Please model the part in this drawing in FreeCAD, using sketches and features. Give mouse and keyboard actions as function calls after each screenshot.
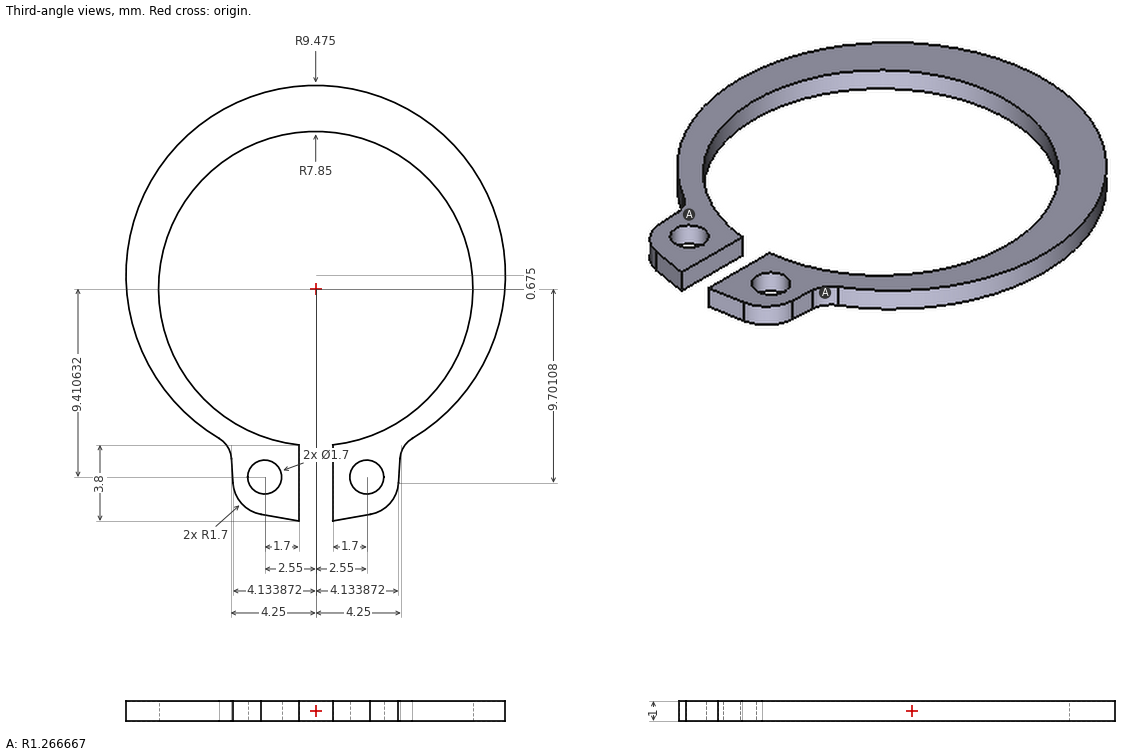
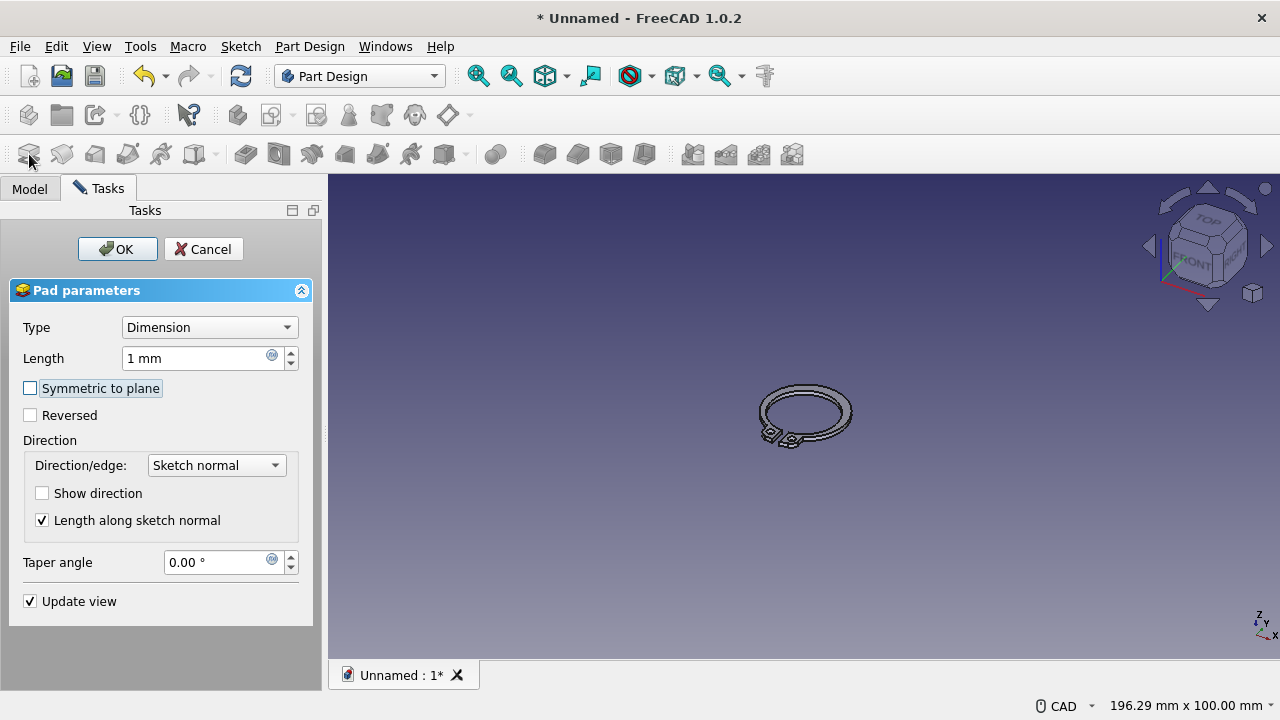
click(31, 388)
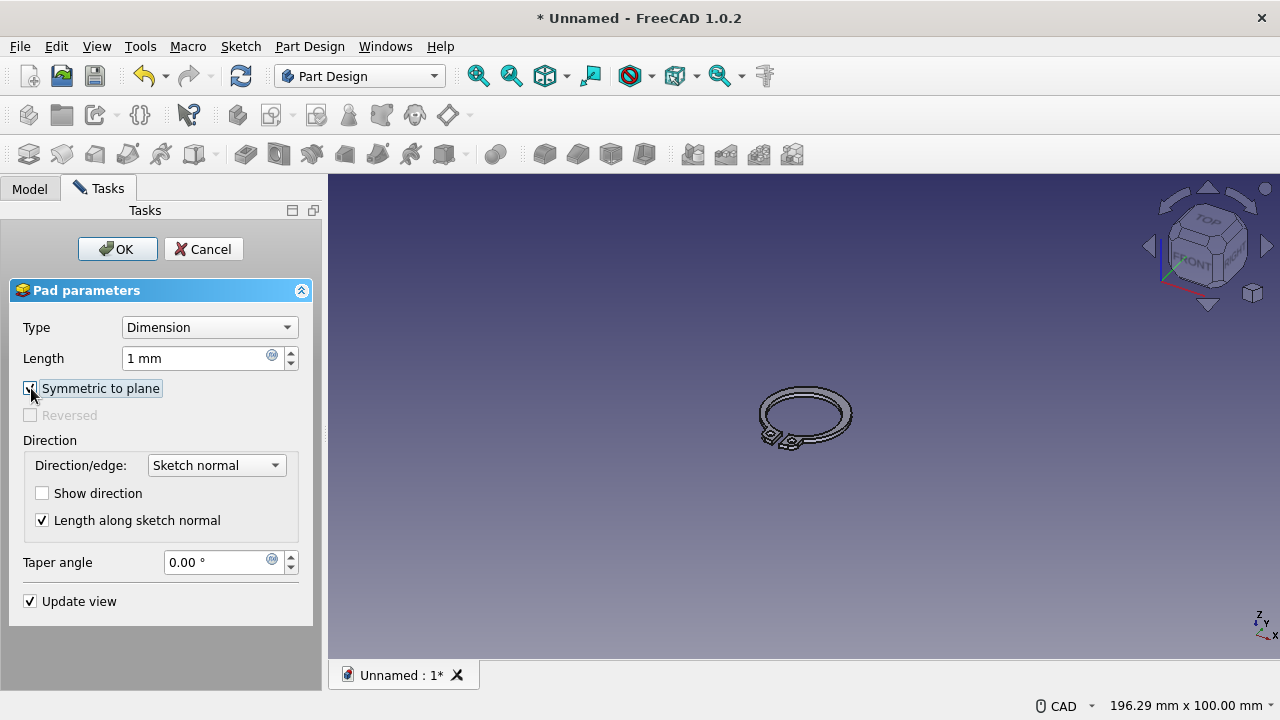
click(118, 249)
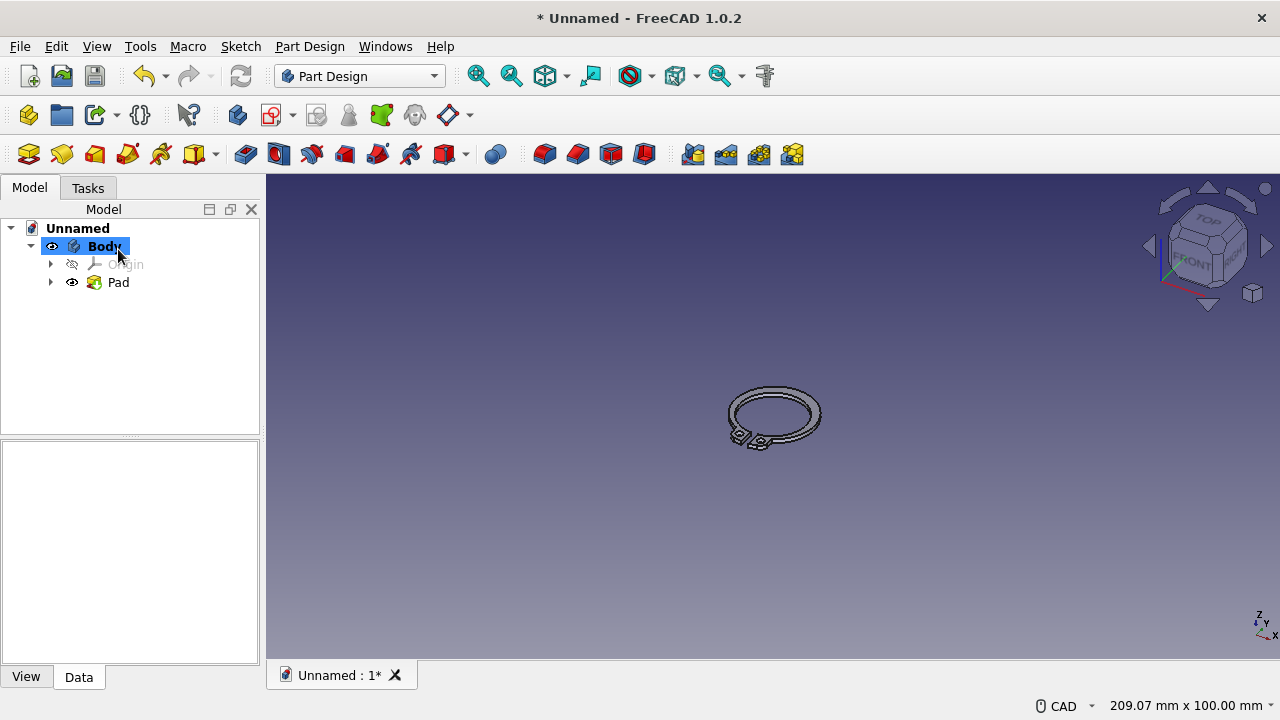
click(479, 76)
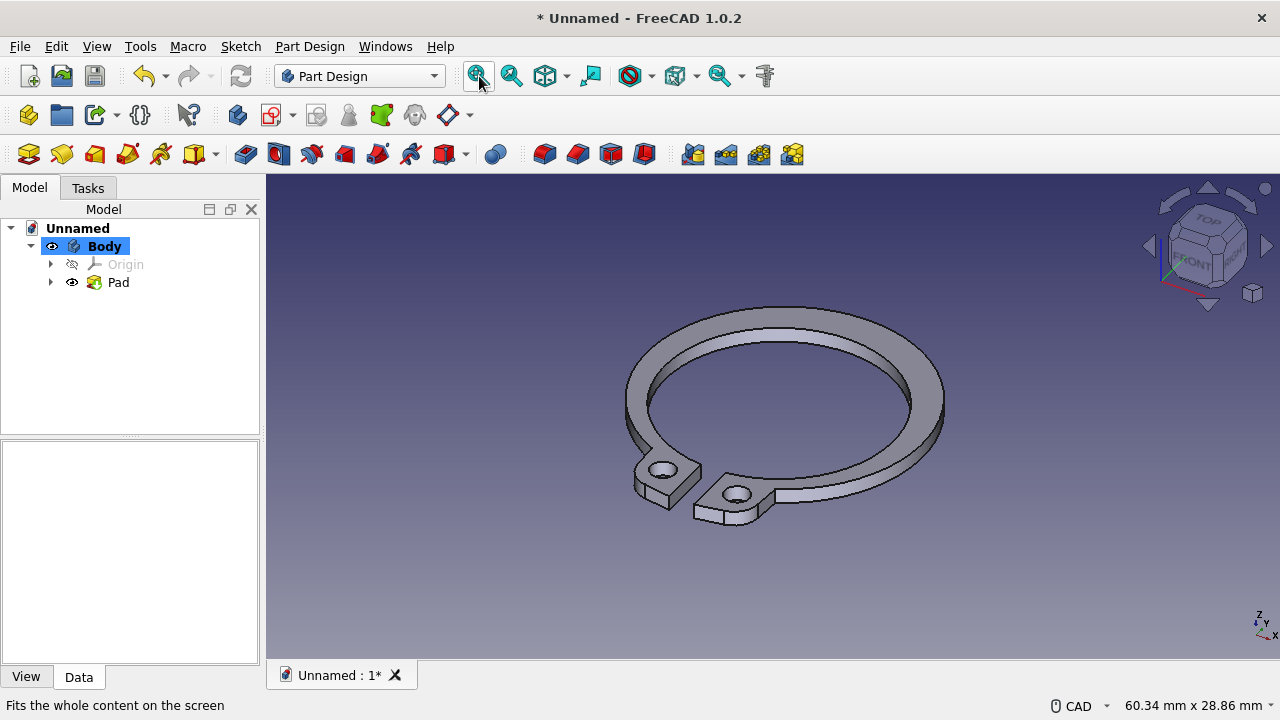
scroll(652, 454, up, 5)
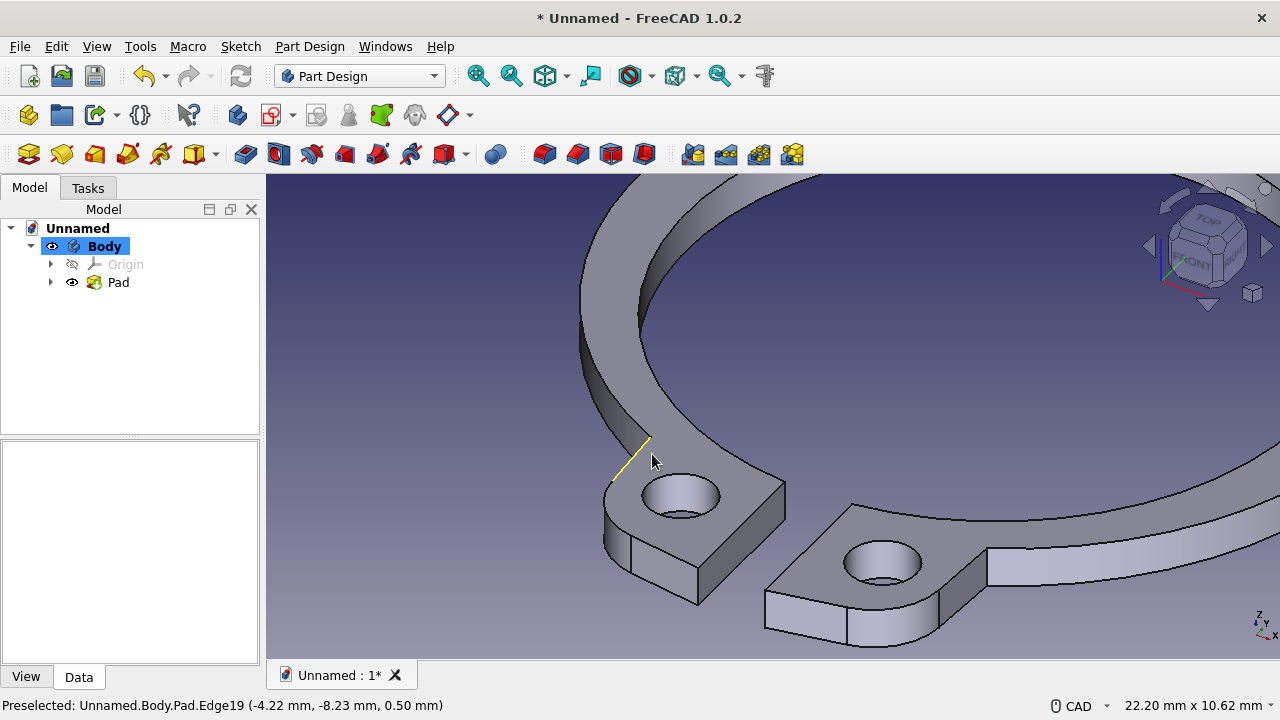
click(479, 76)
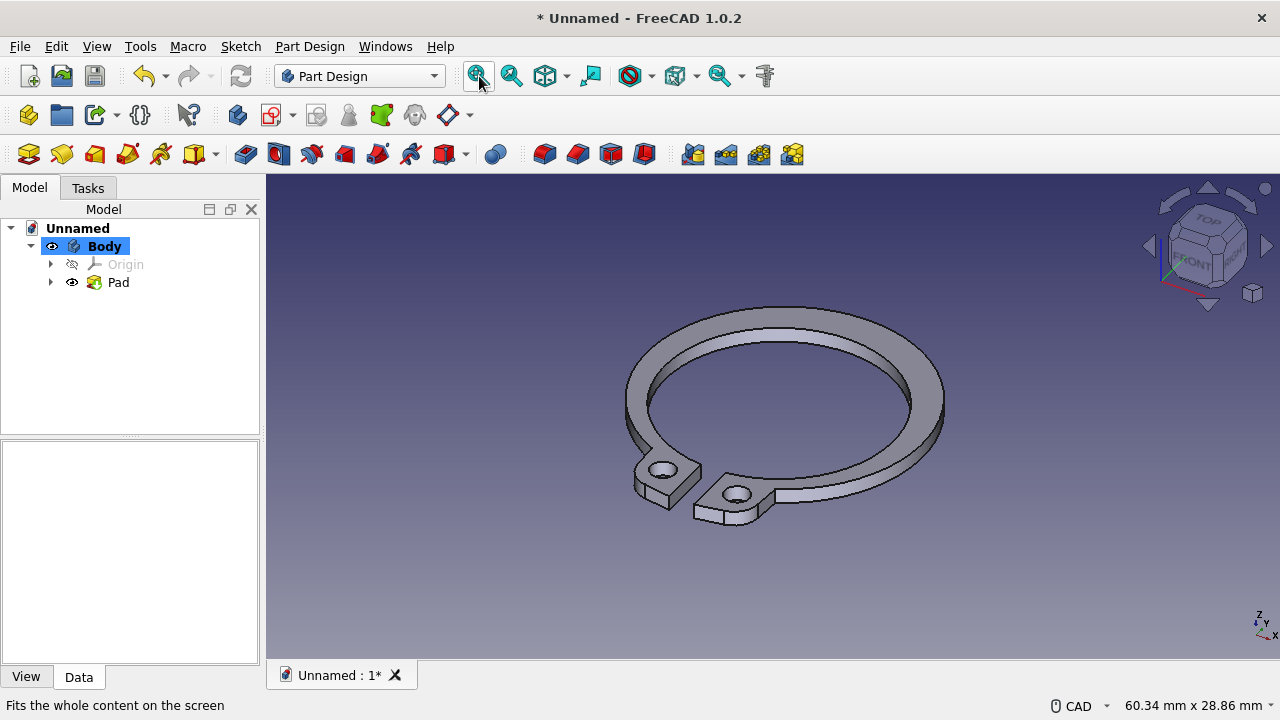
key(0)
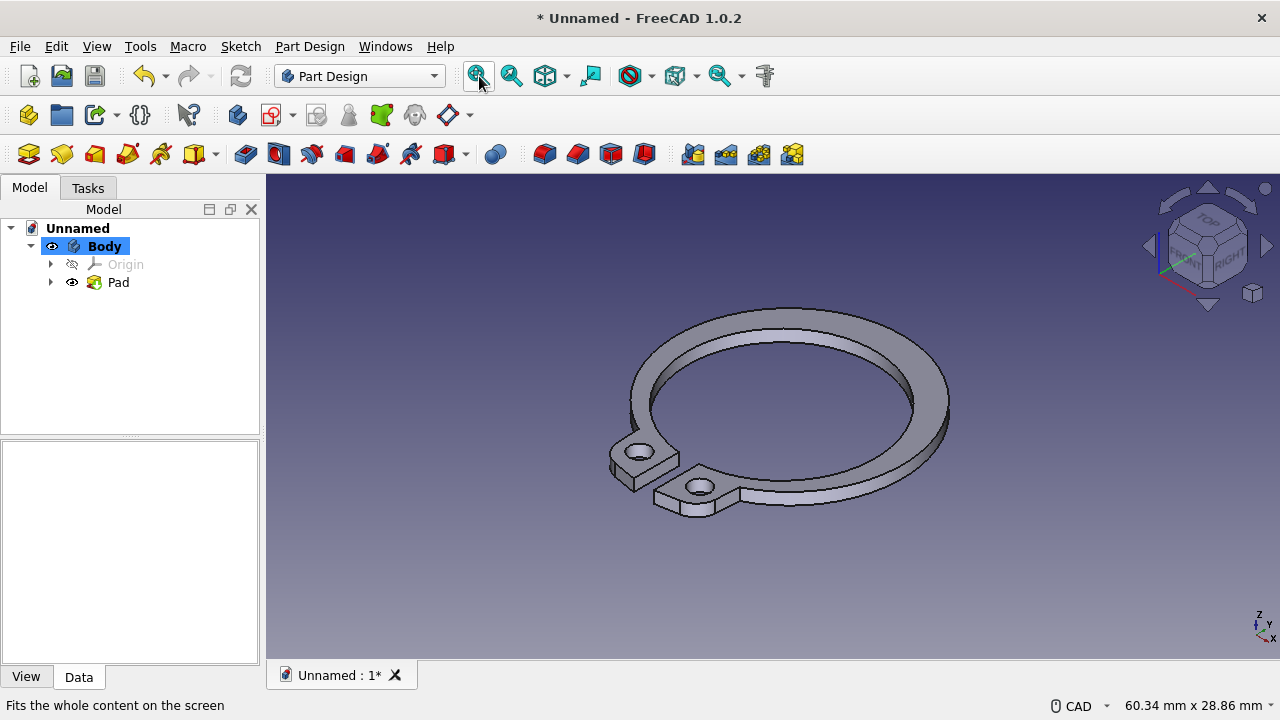
scroll(639, 435, up, 5)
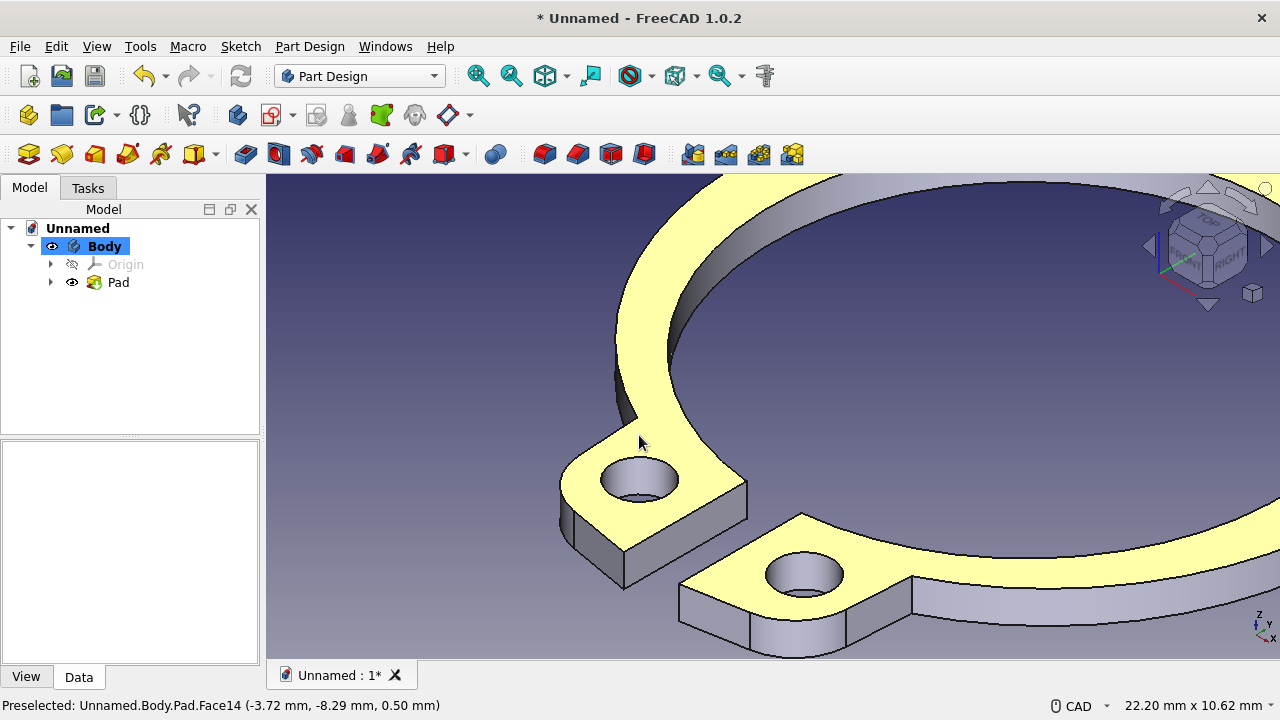
click(479, 76)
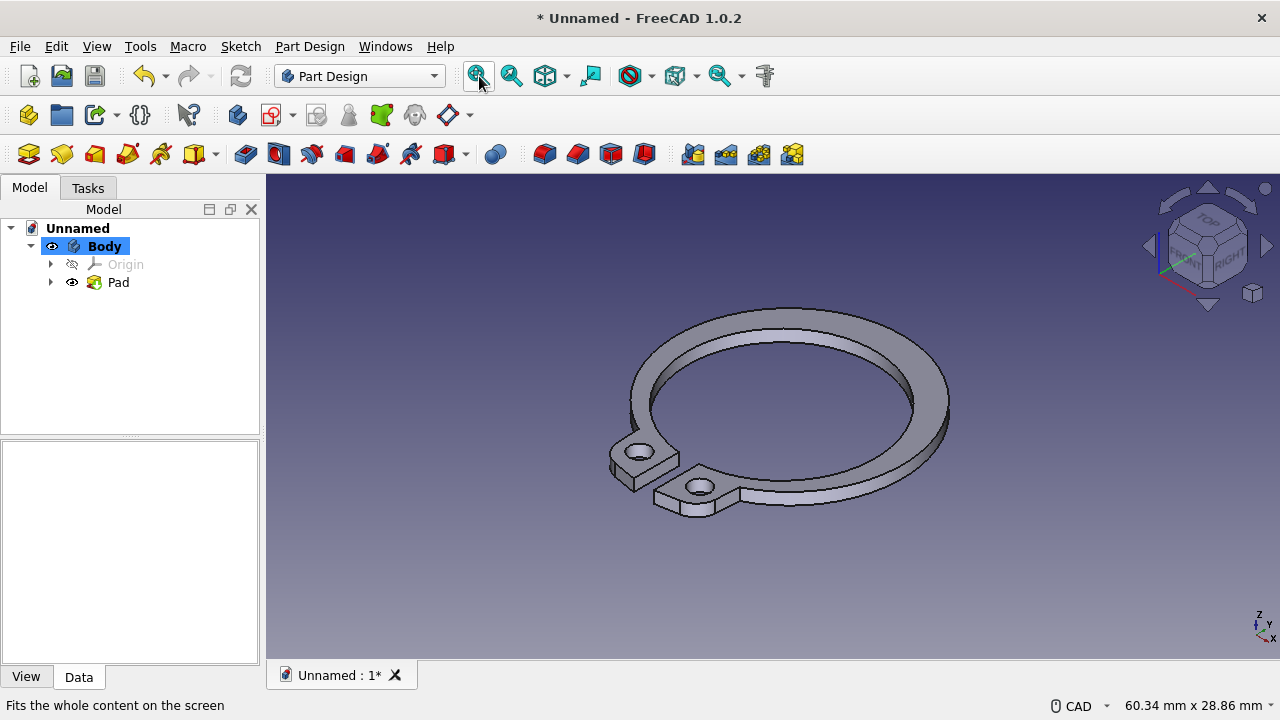
key(2)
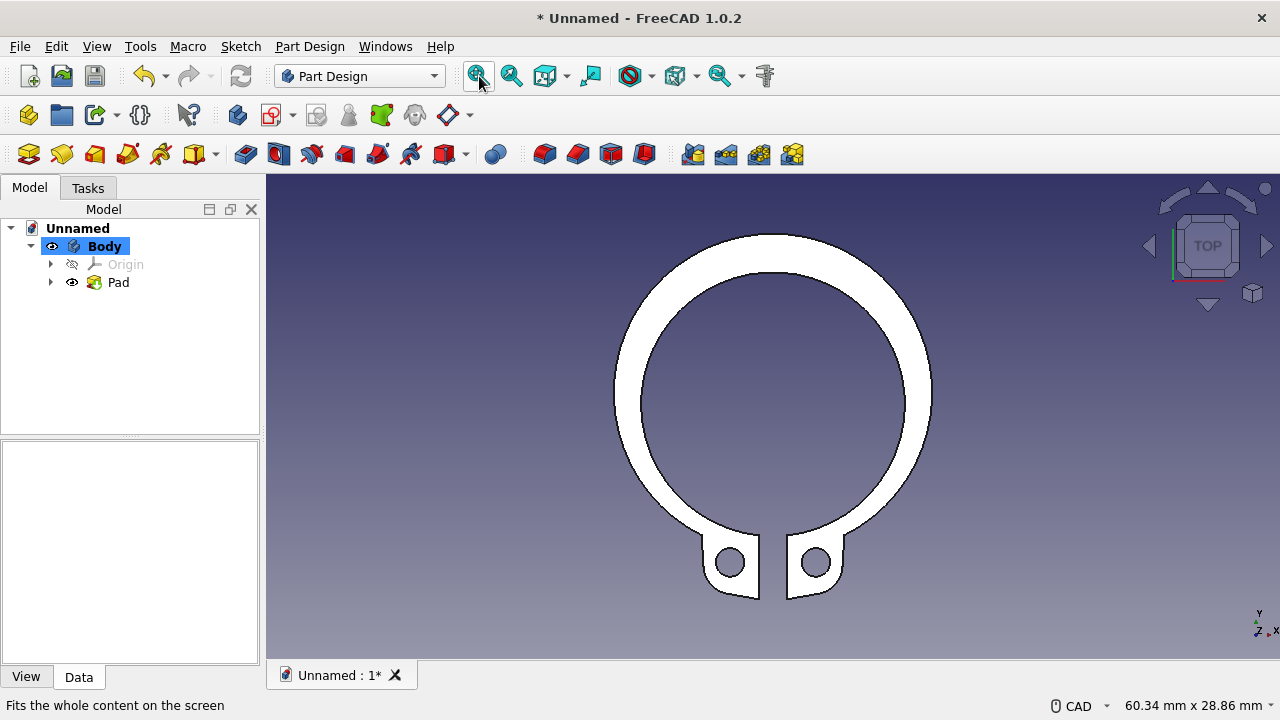
scroll(702, 534, up, 5)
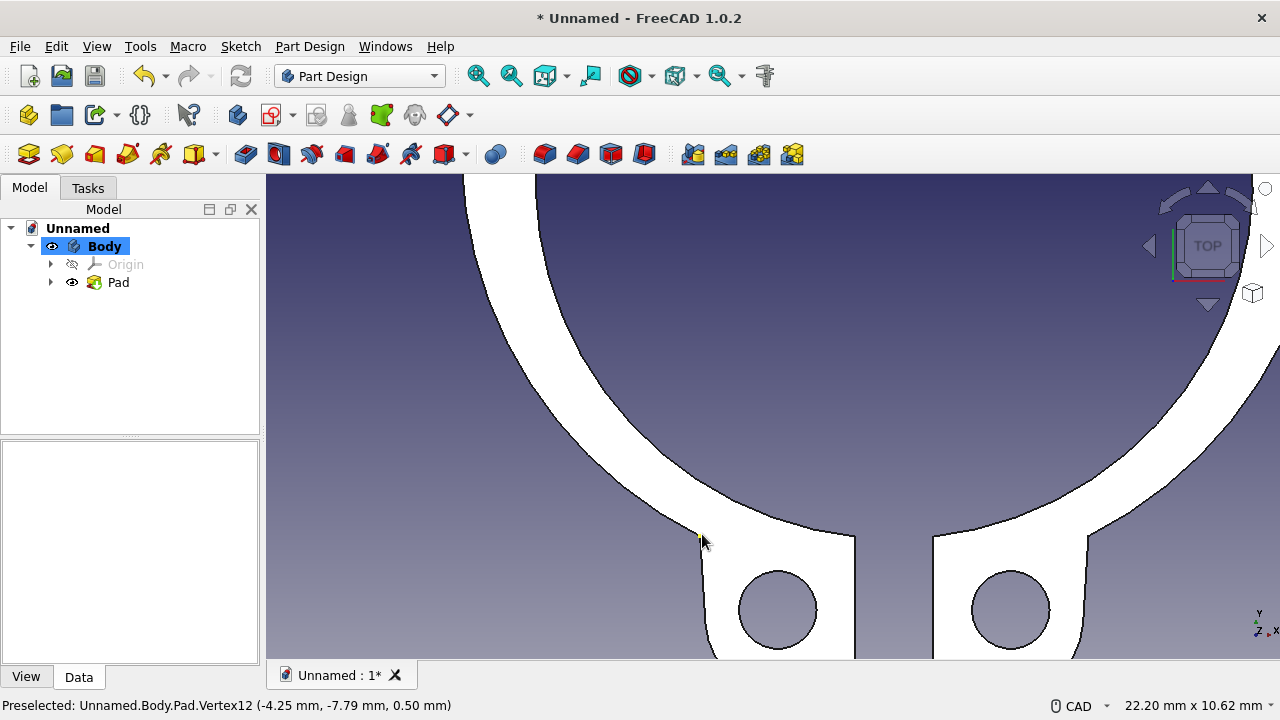
click(479, 76)